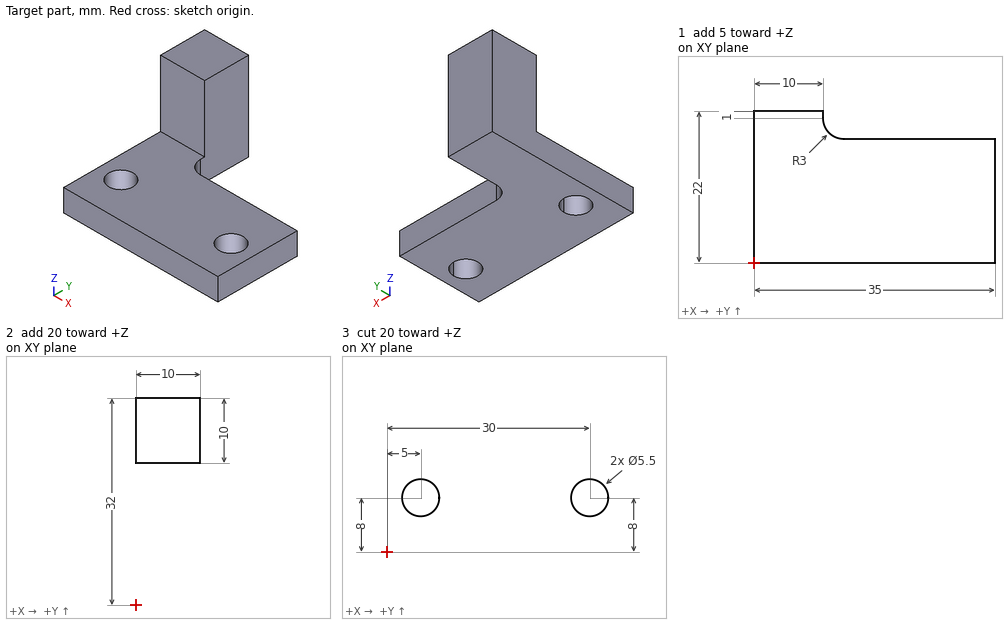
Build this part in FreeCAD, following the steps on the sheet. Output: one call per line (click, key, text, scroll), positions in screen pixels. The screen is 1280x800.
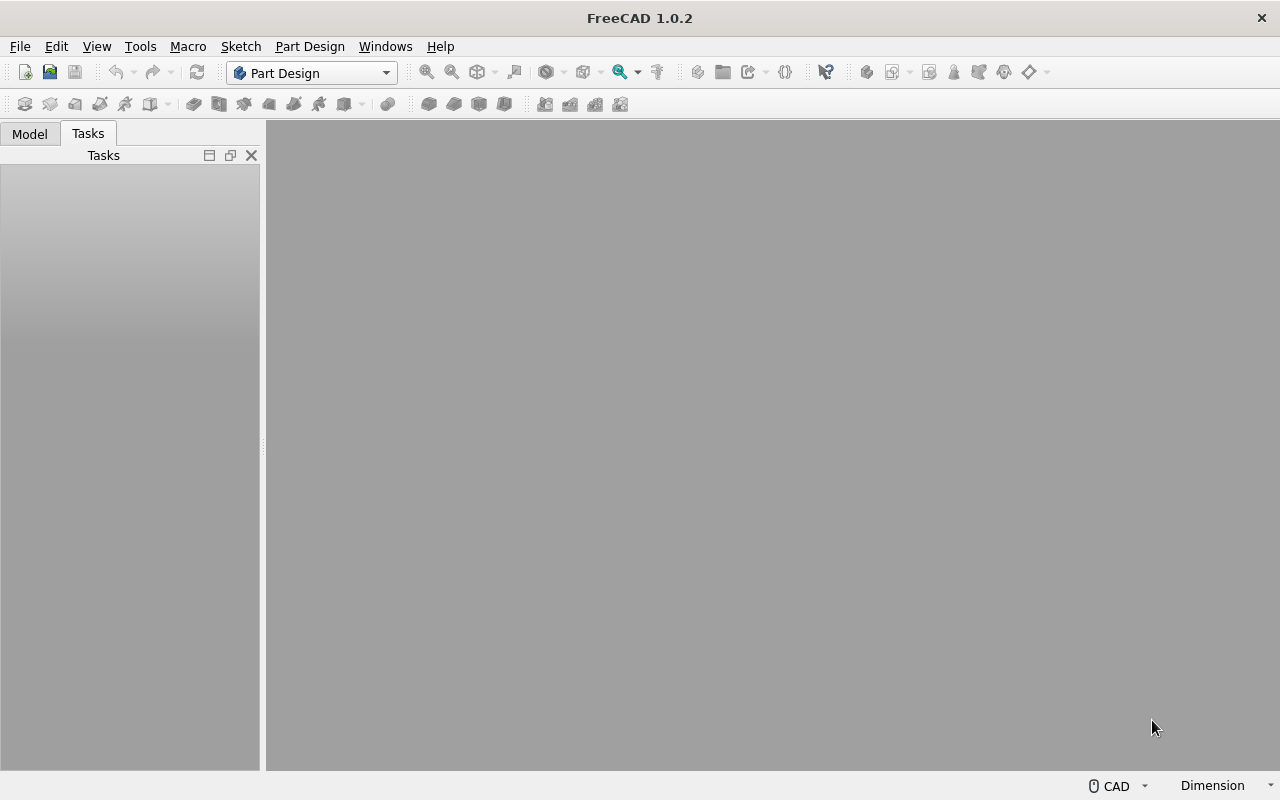
click(25, 72)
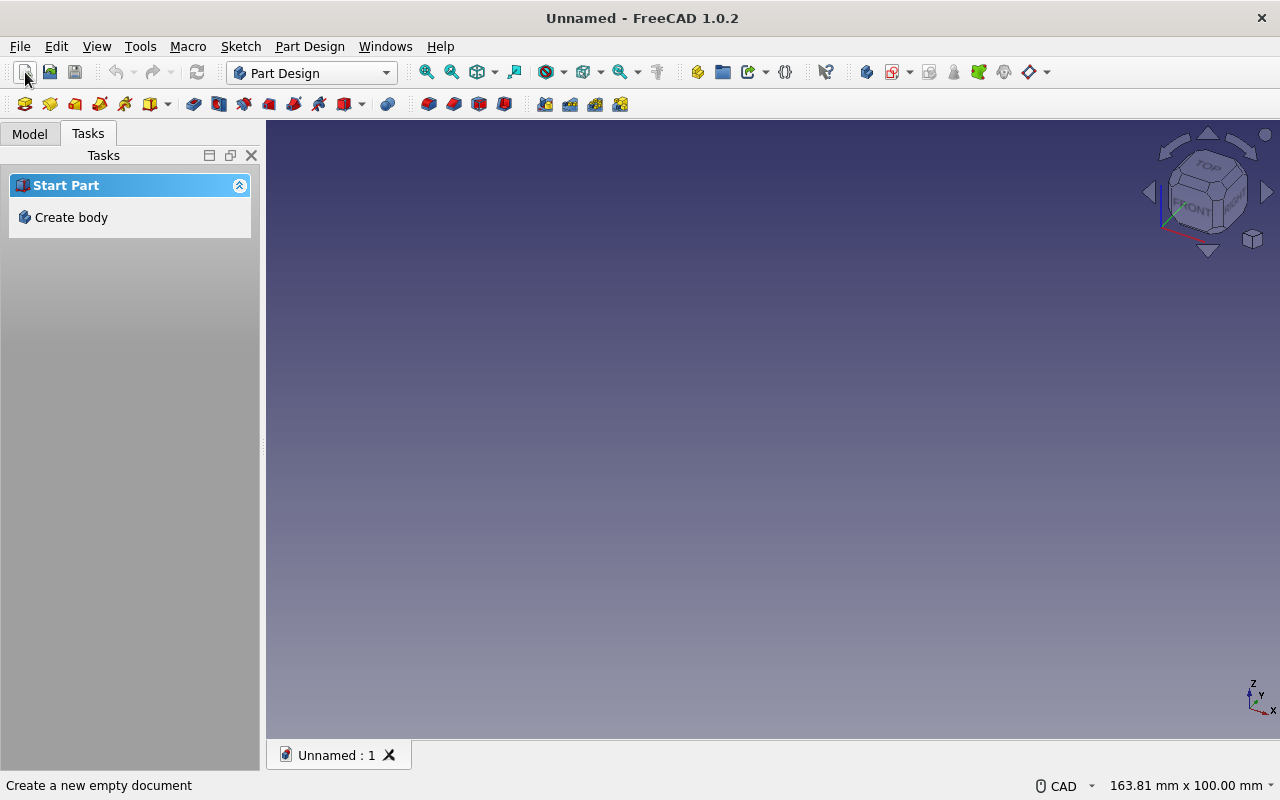
click(892, 72)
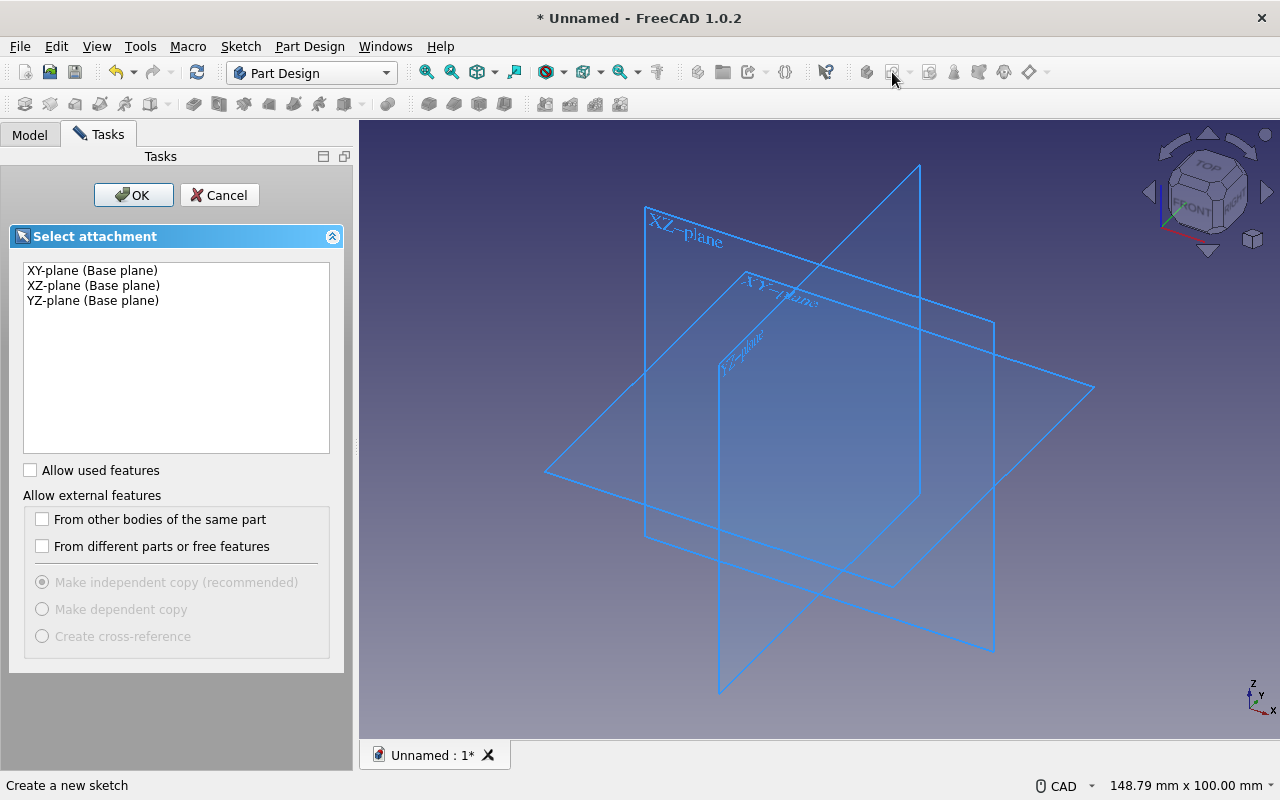
click(84, 270)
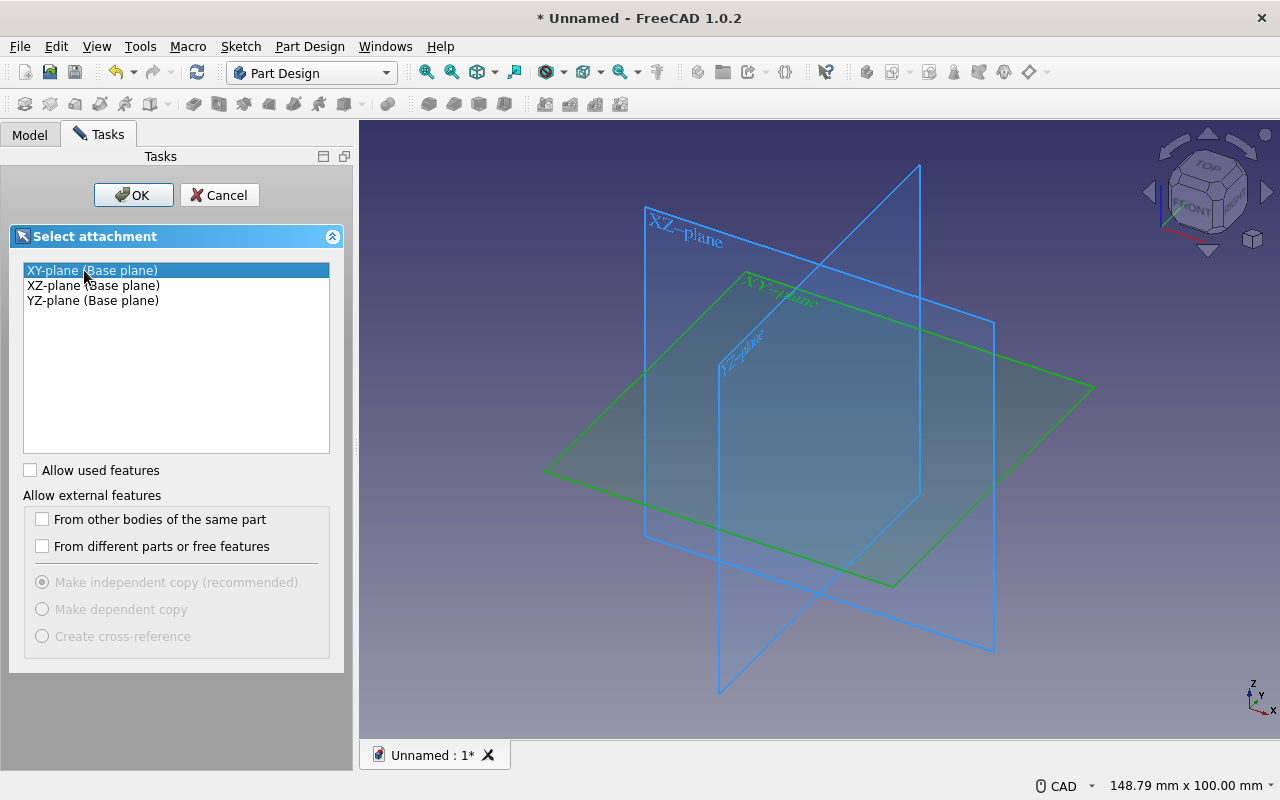
click(134, 195)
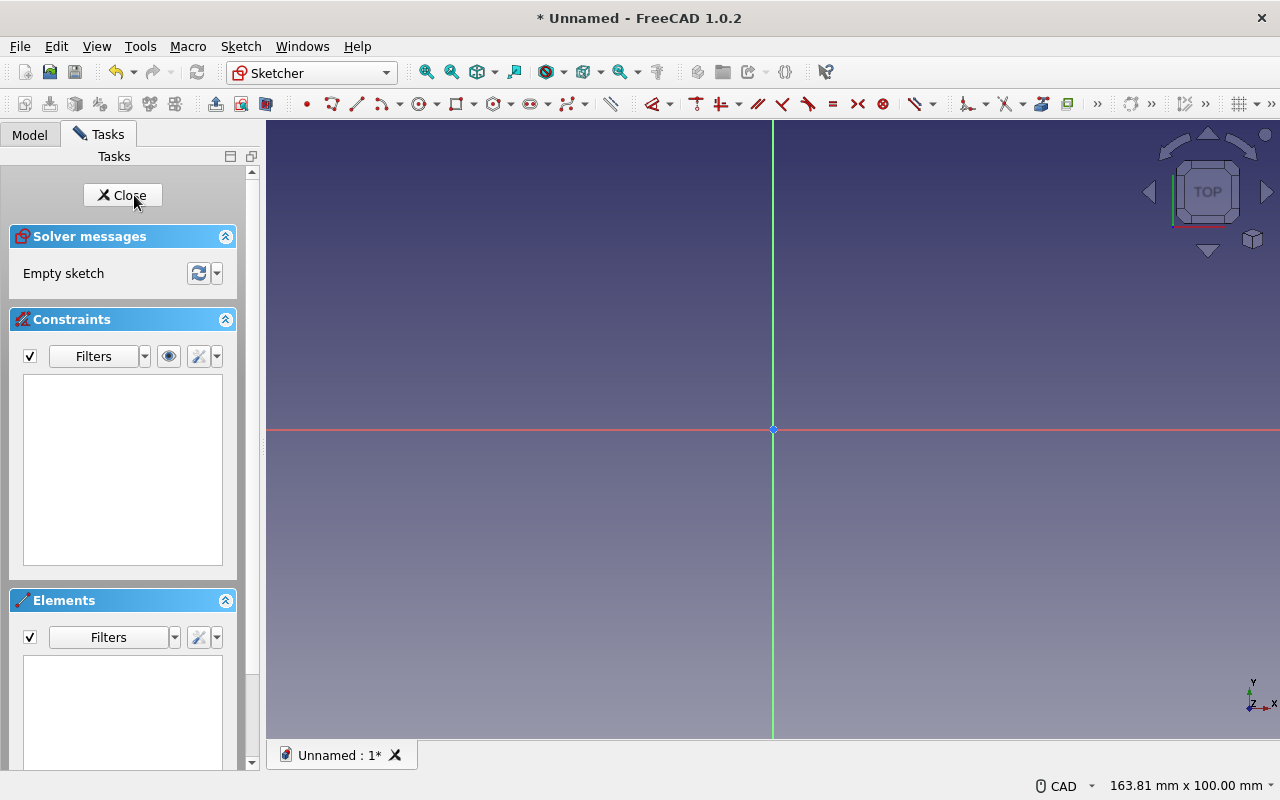
scroll(984, 322, up, 5)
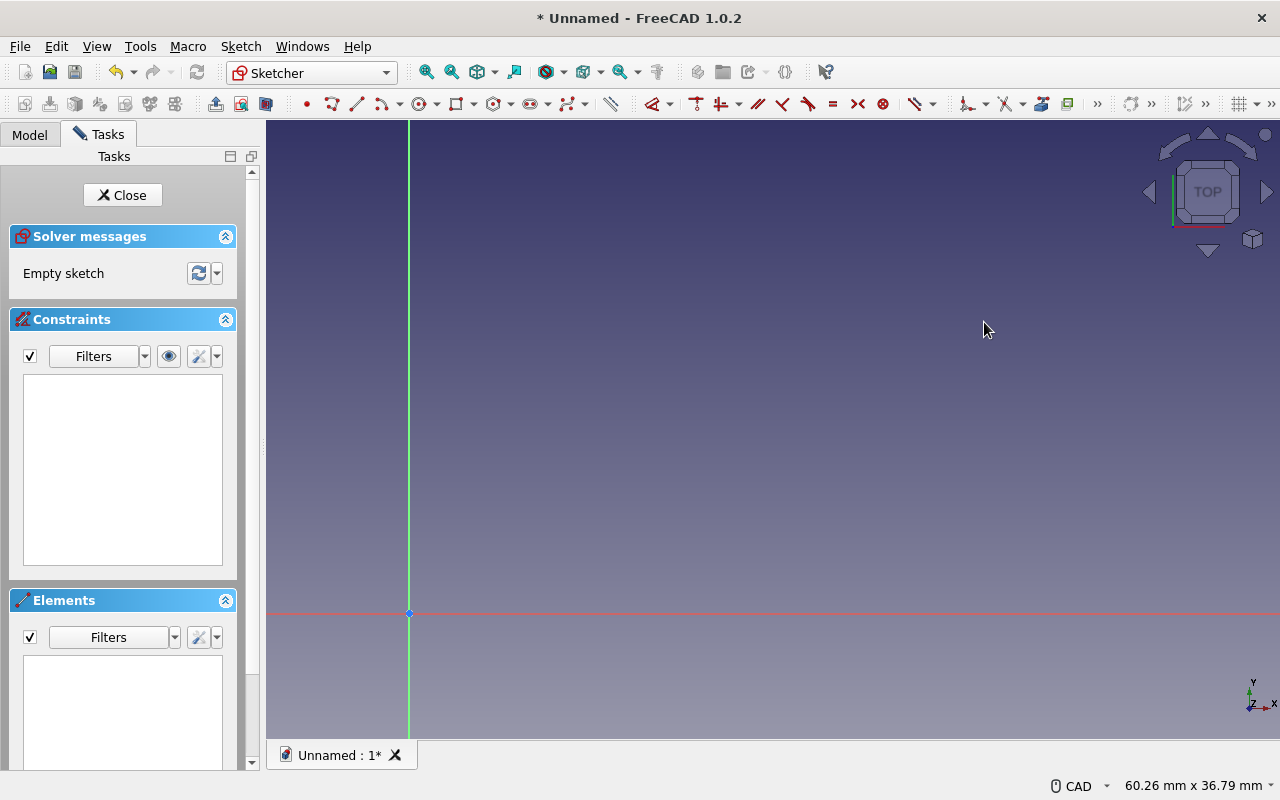
click(332, 104)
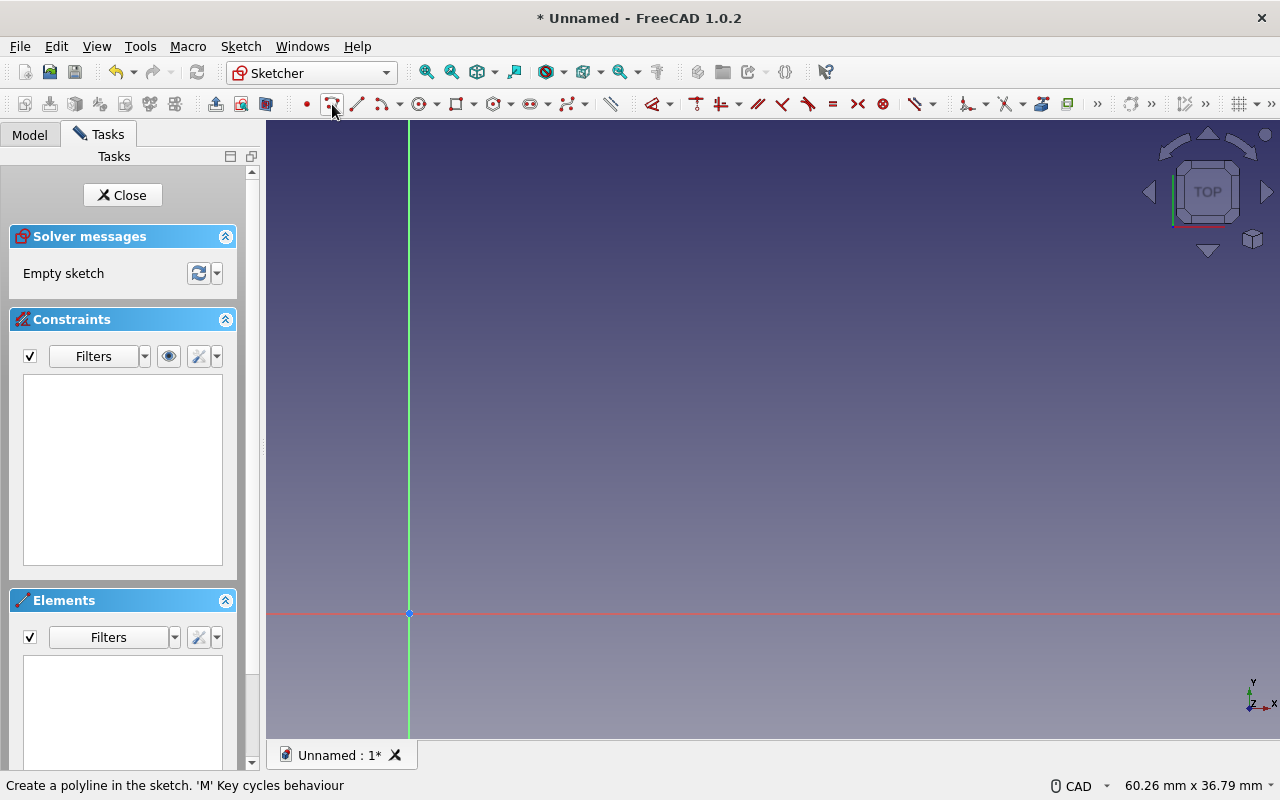
click(577, 260)
click(577, 243)
click(409, 243)
click(409, 614)
click(998, 605)
click(998, 311)
click(628, 311)
right_click(628, 311)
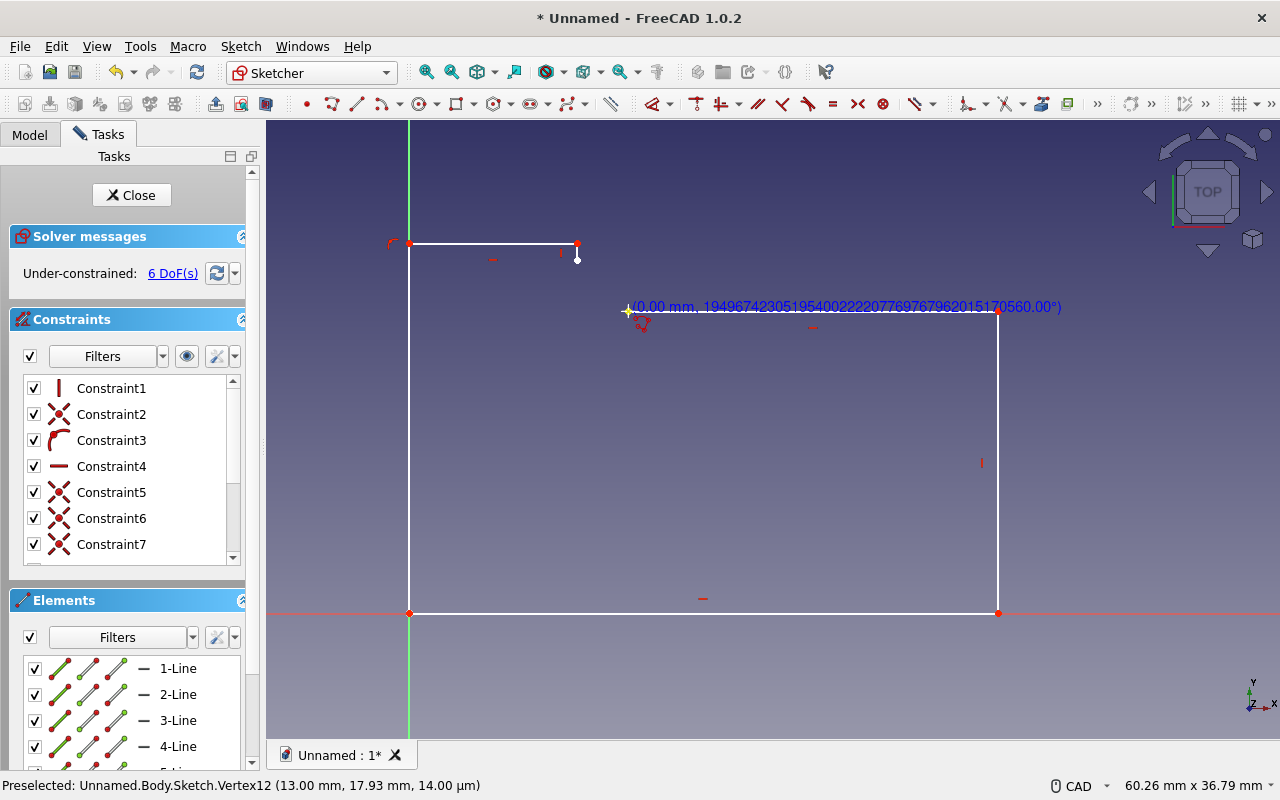
key(g)
key(3)
key(a)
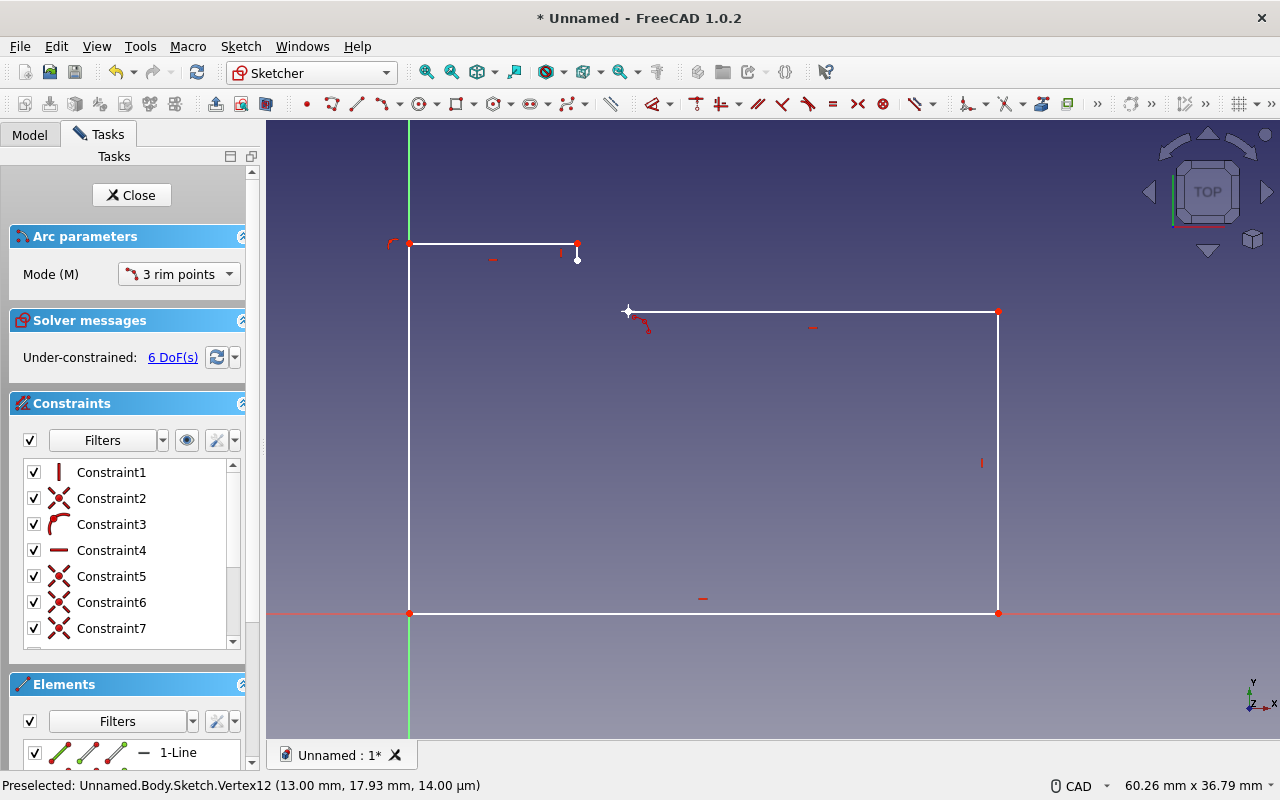
click(628, 312)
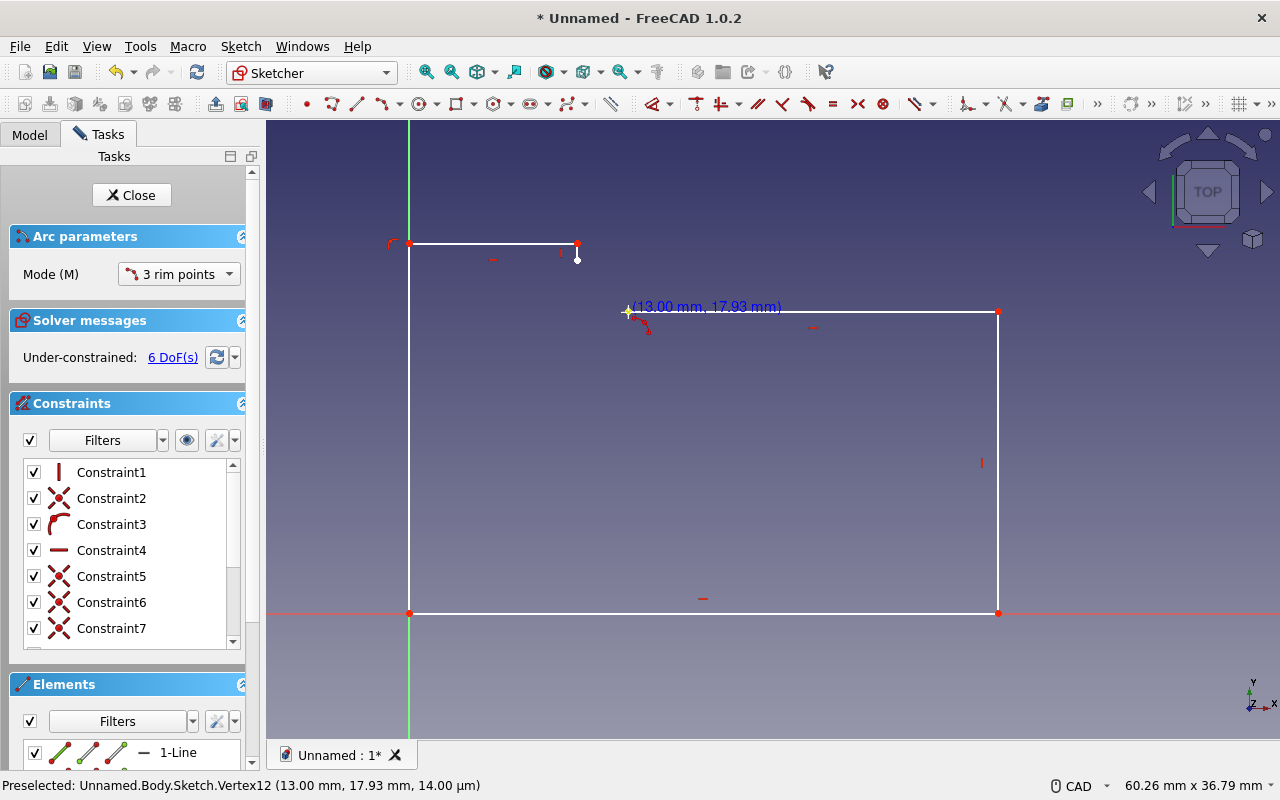
scroll(577, 260, up, 4)